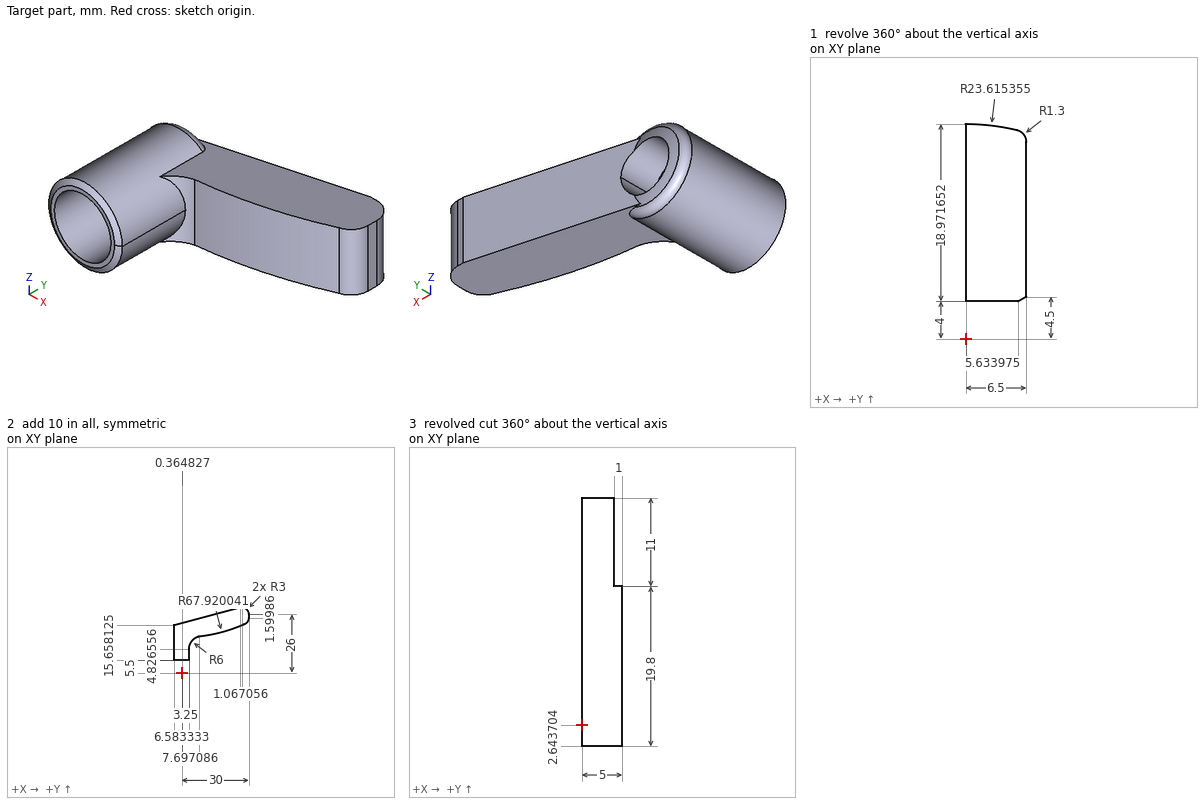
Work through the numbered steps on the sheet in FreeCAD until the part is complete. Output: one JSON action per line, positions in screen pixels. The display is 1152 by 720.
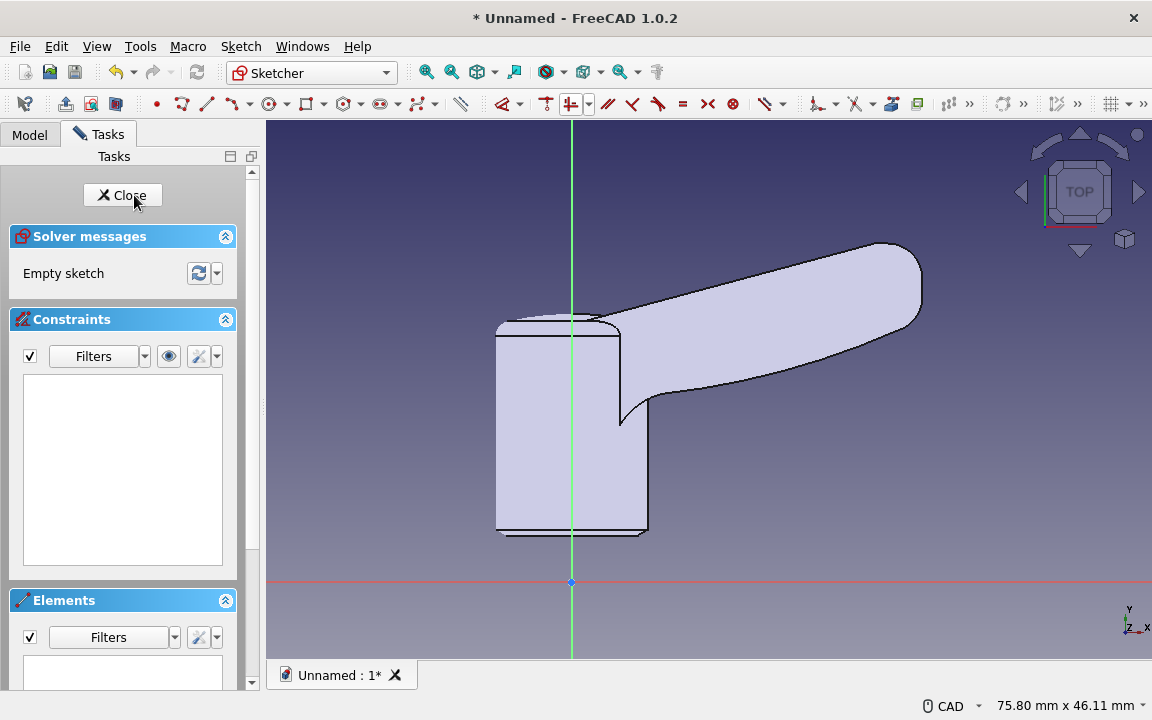
{"action": "scroll", "coordinate": [819, 192], "scroll_direction": "down", "scroll_amount": 1}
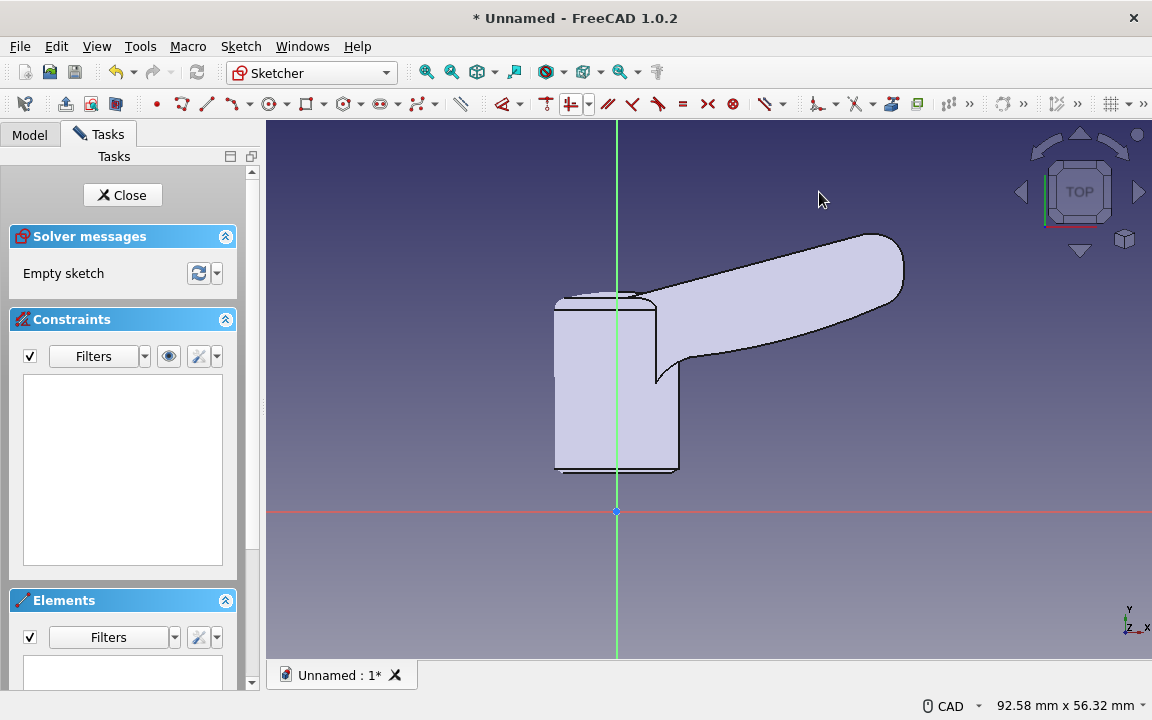
{"action": "left_click", "coordinate": [182, 104]}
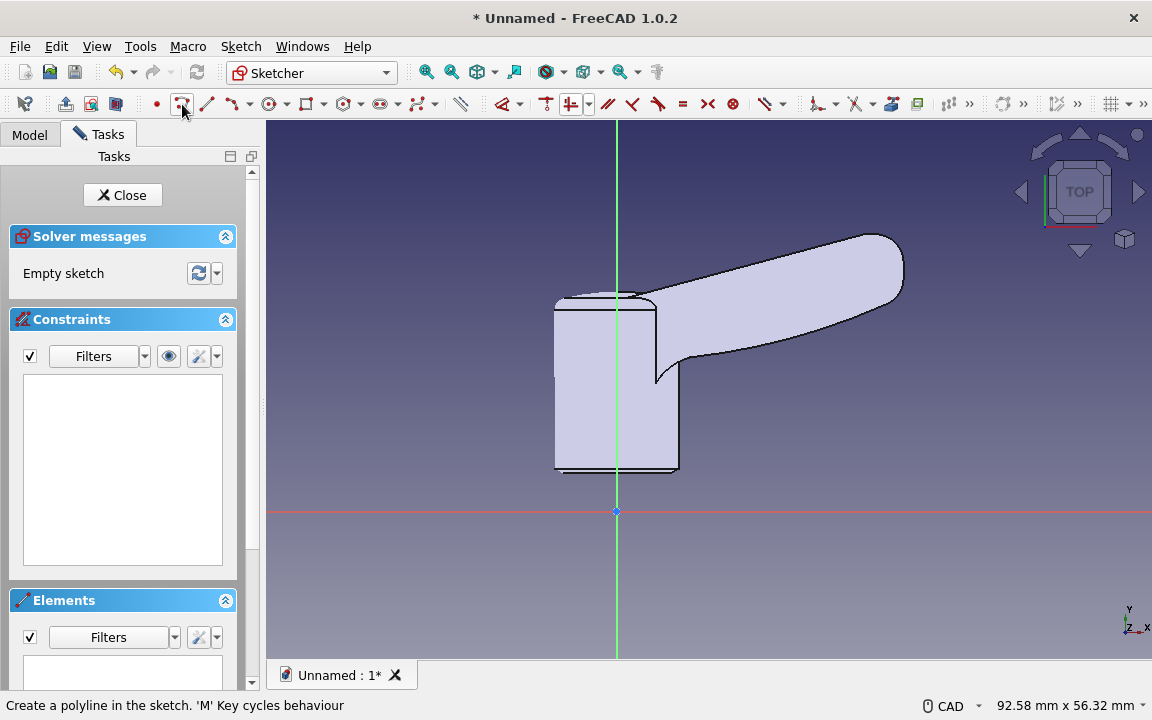
{"action": "left_click", "coordinate": [617, 537]}
{"action": "left_click", "coordinate": [664, 537]}
{"action": "left_click", "coordinate": [664, 347]}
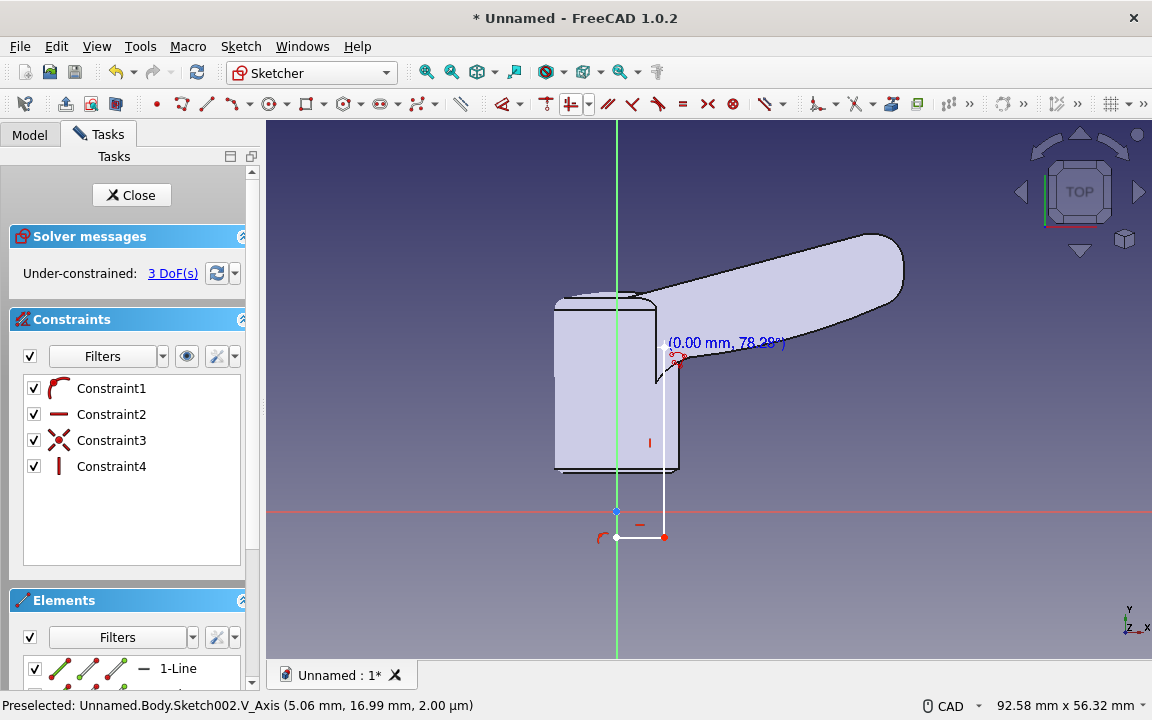
{"action": "scroll", "coordinate": [655, 347], "scroll_direction": "up", "scroll_amount": 3}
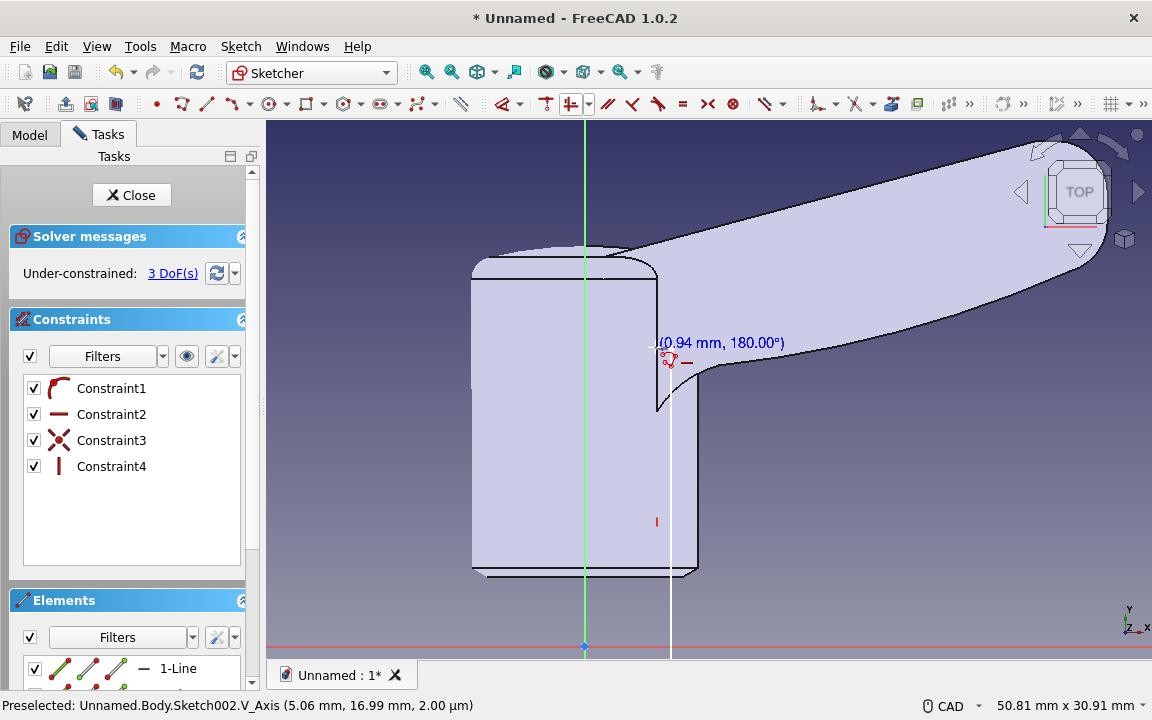
{"action": "left_click", "coordinate": [654, 347]}
{"action": "left_click", "coordinate": [654, 156]}
{"action": "left_click", "coordinate": [594, 156]}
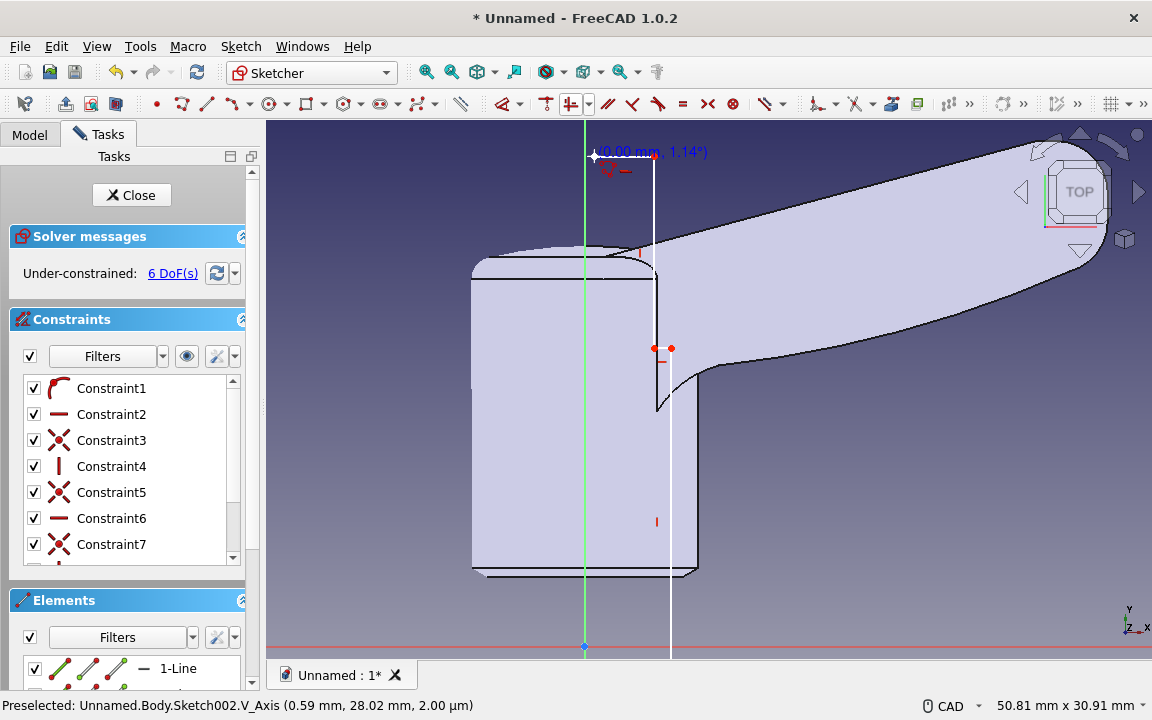
{"action": "scroll", "coordinate": [665, 319], "scroll_direction": "down", "scroll_amount": 2}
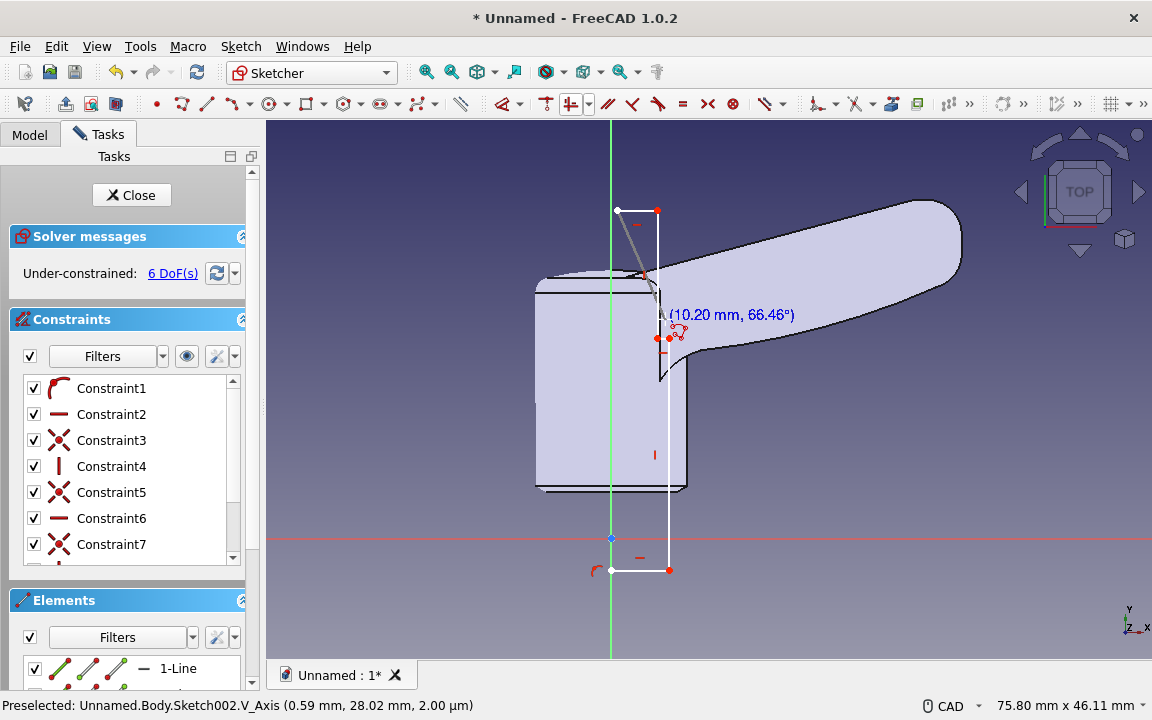
{"action": "left_click", "coordinate": [611, 571]}
{"action": "key", "text": "Escape"}
{"action": "key", "text": "Escape"}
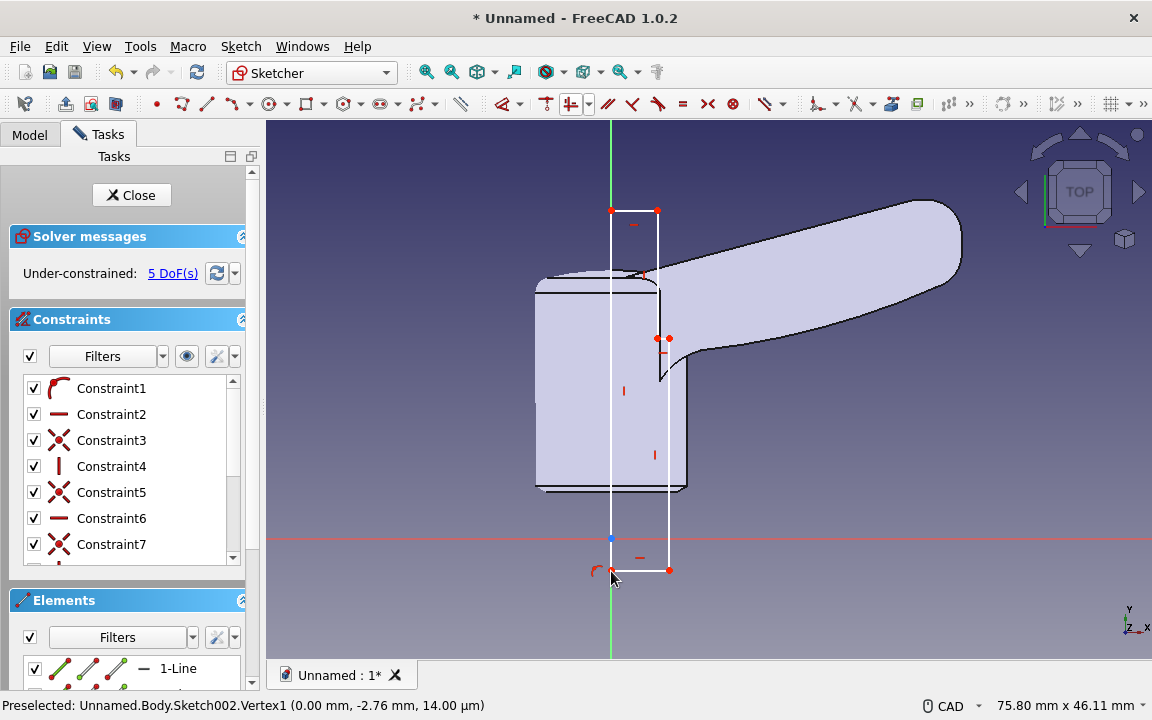
{"action": "left_click", "coordinate": [502, 104]}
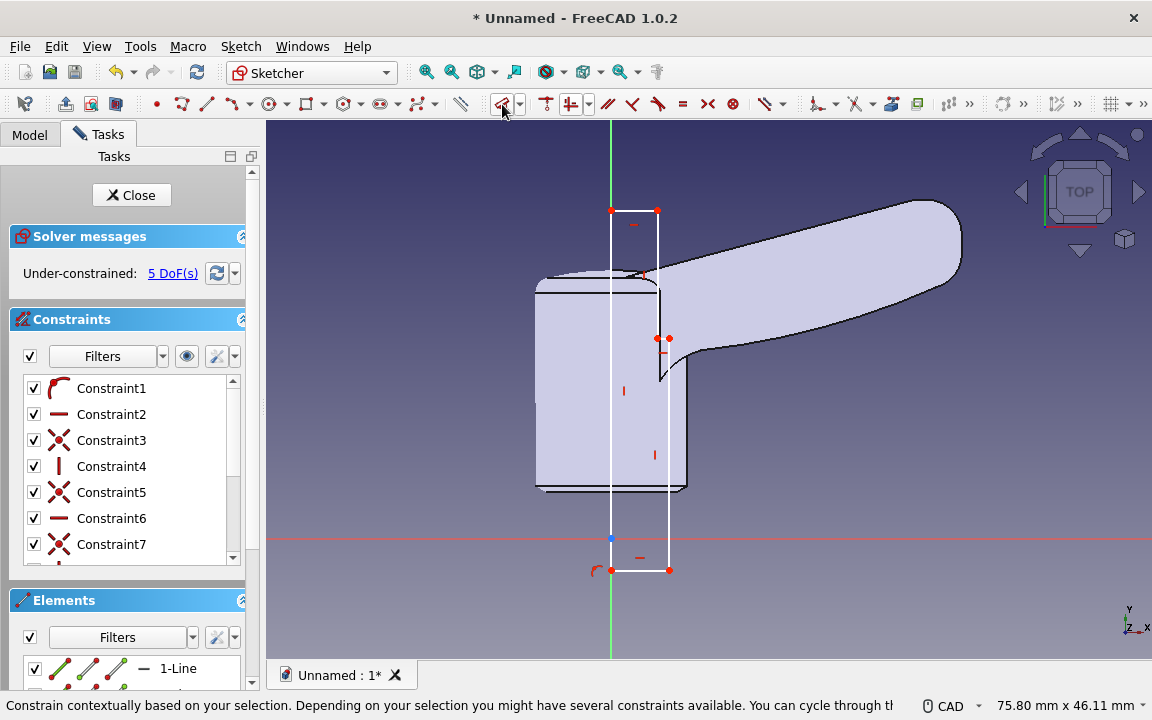
{"action": "left_click", "coordinate": [629, 571]}
{"action": "left_click", "coordinate": [640, 605]}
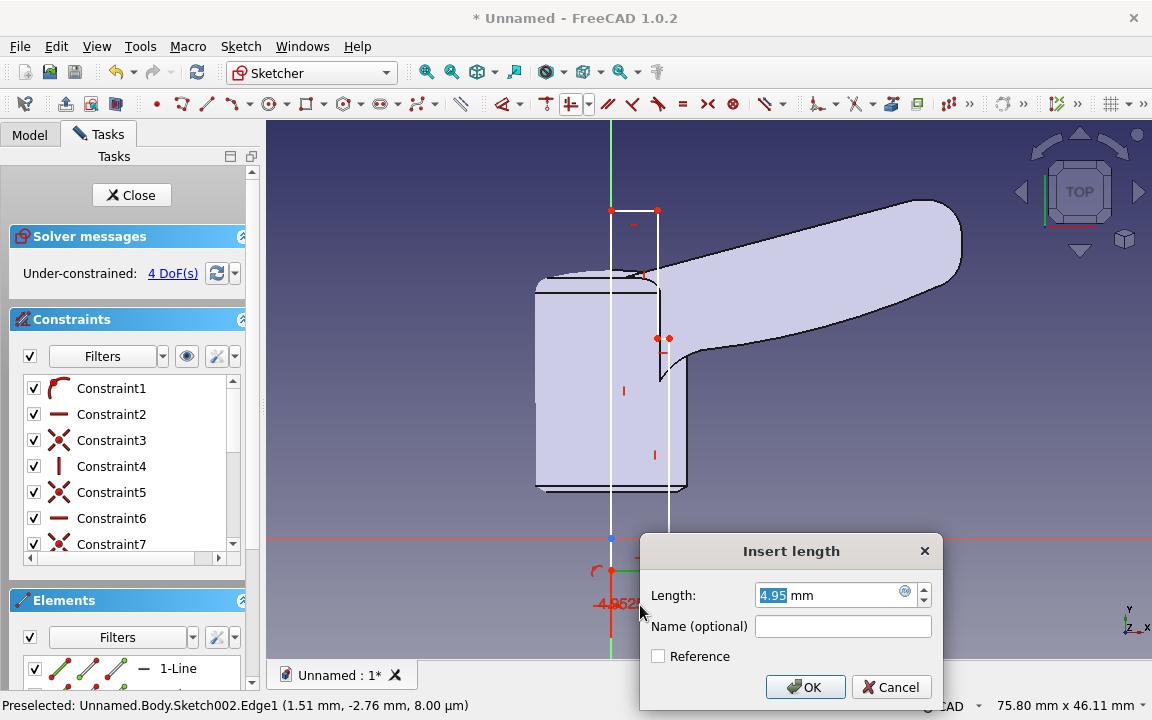
{"action": "type", "text": "5"}
{"action": "key", "text": "Return"}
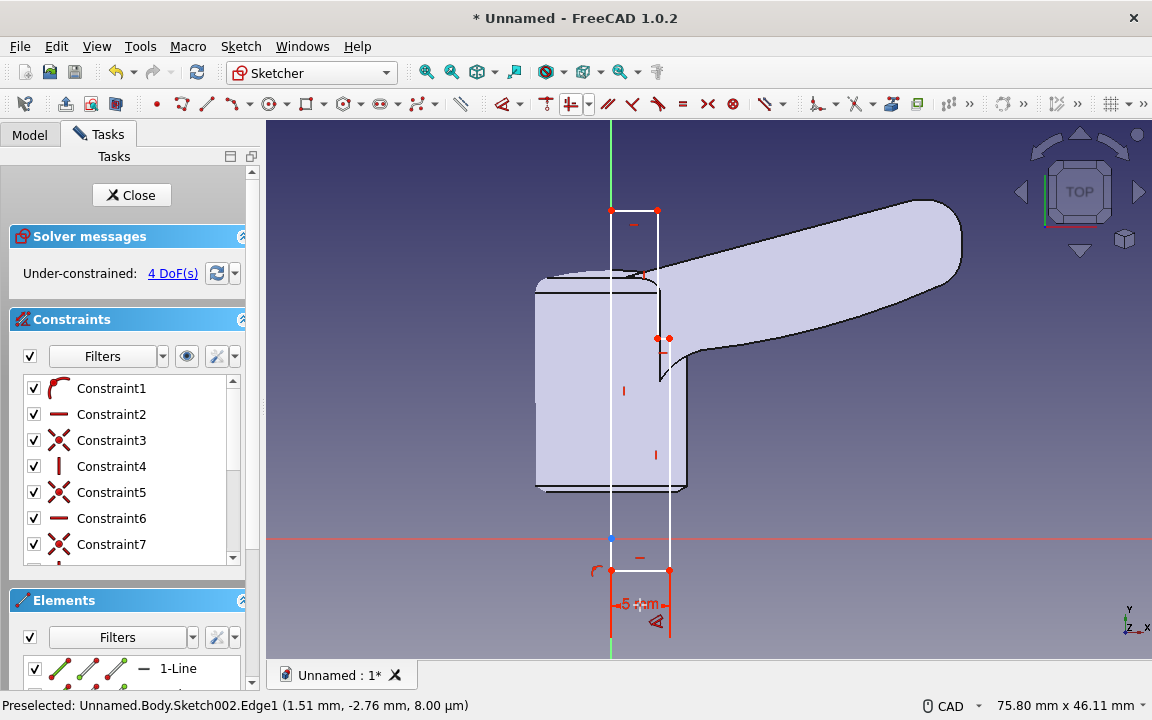
{"action": "scroll", "coordinate": [664, 339], "scroll_direction": "up", "scroll_amount": 7}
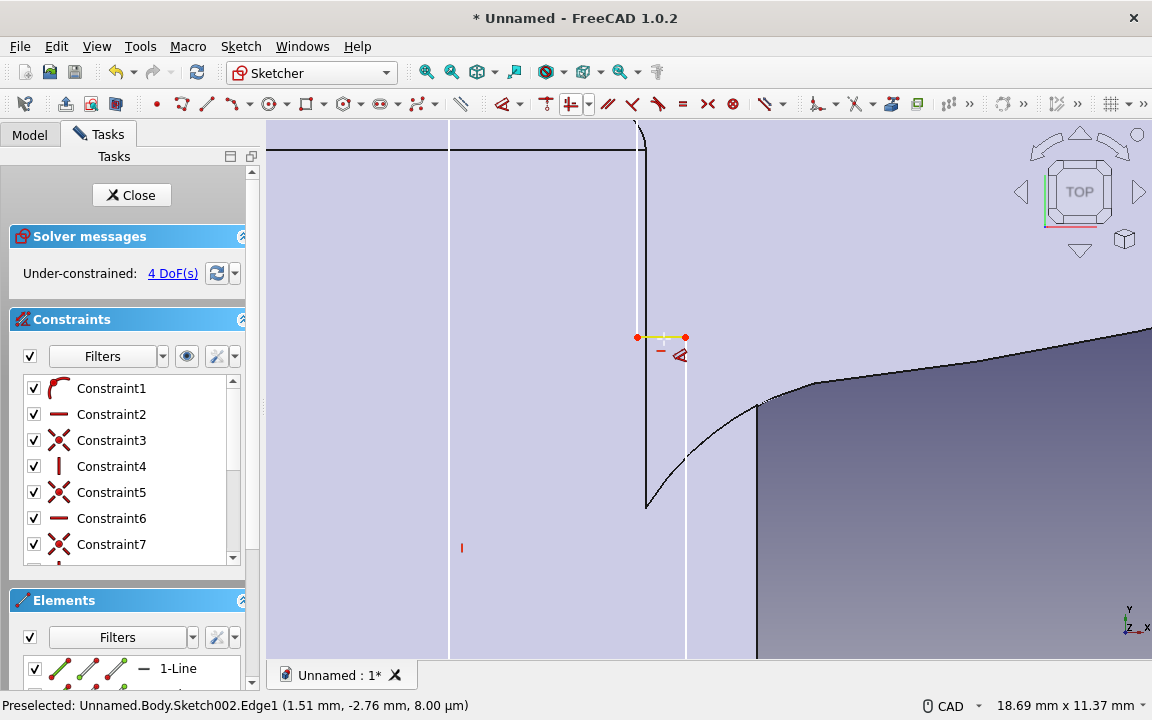
{"action": "left_click", "coordinate": [662, 337]}
{"action": "left_click", "coordinate": [662, 303]}